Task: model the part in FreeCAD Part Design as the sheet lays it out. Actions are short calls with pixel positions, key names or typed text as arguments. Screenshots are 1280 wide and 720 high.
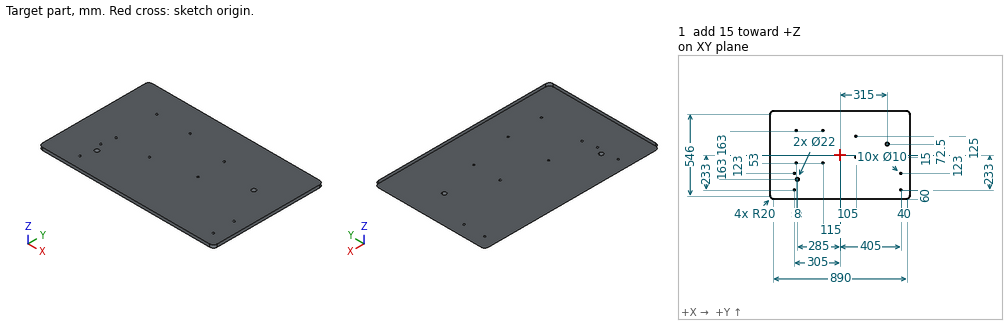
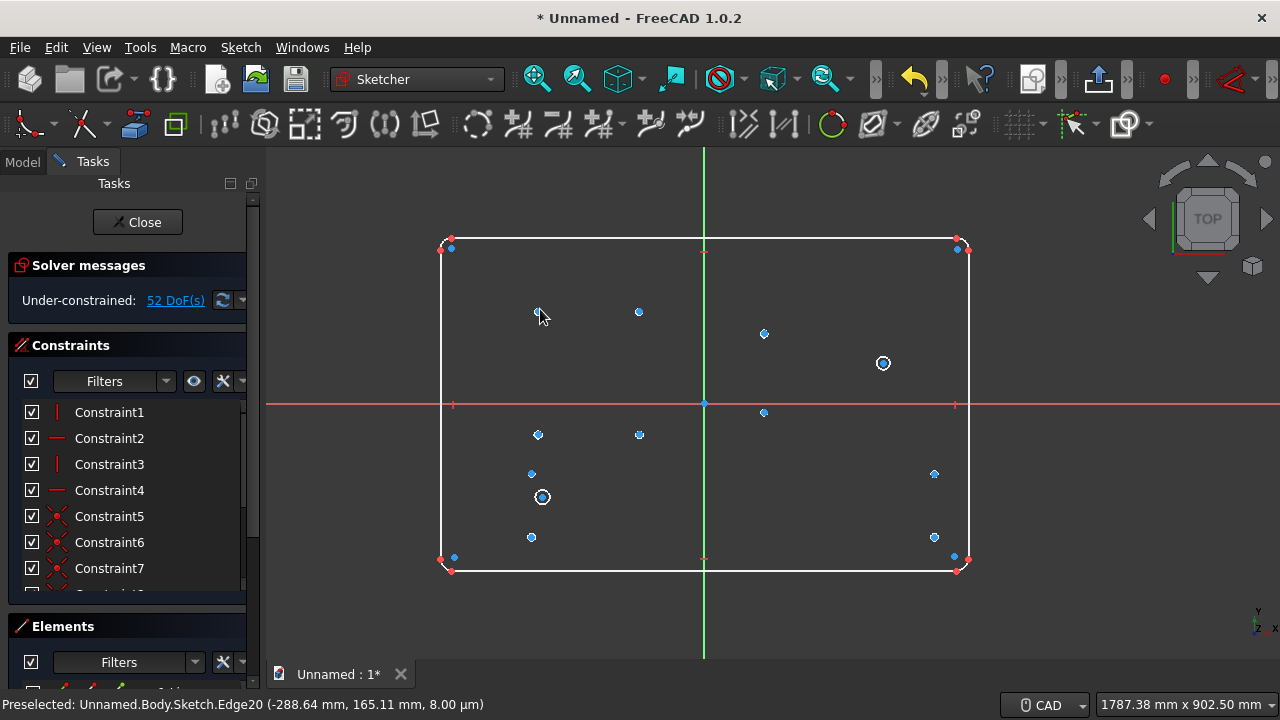
click(441, 343)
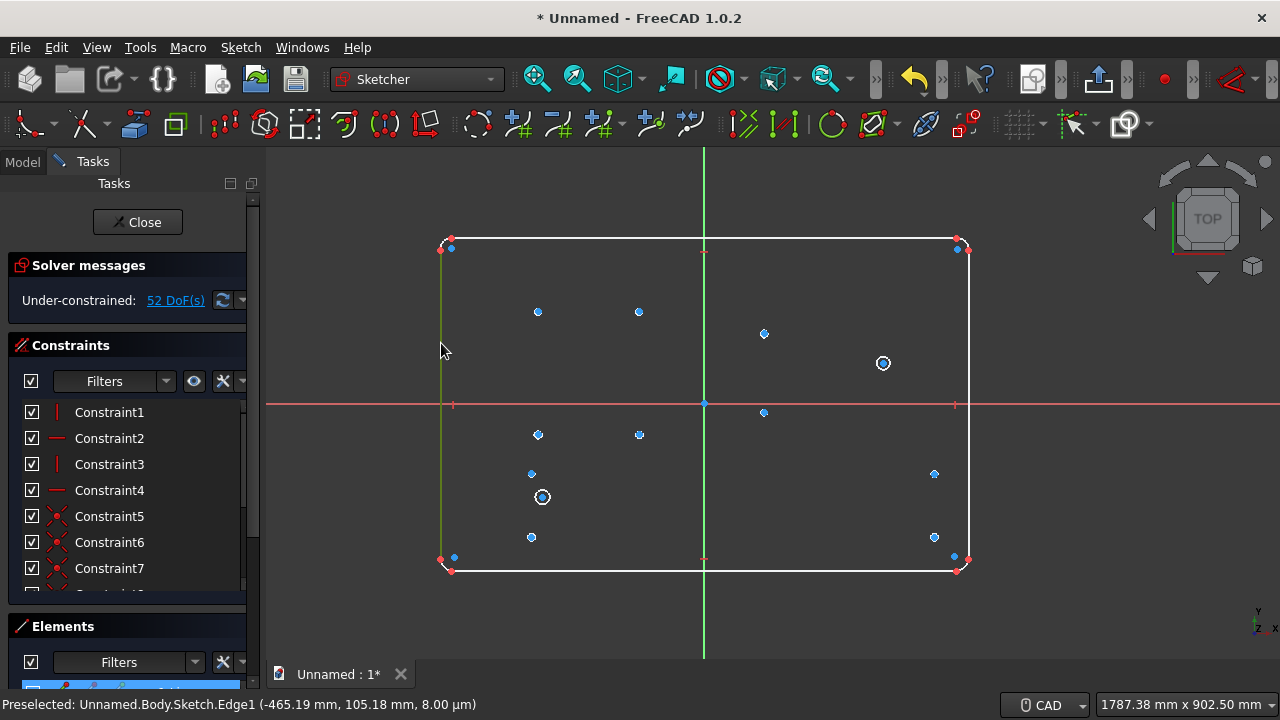
scroll(444, 567, up, 3)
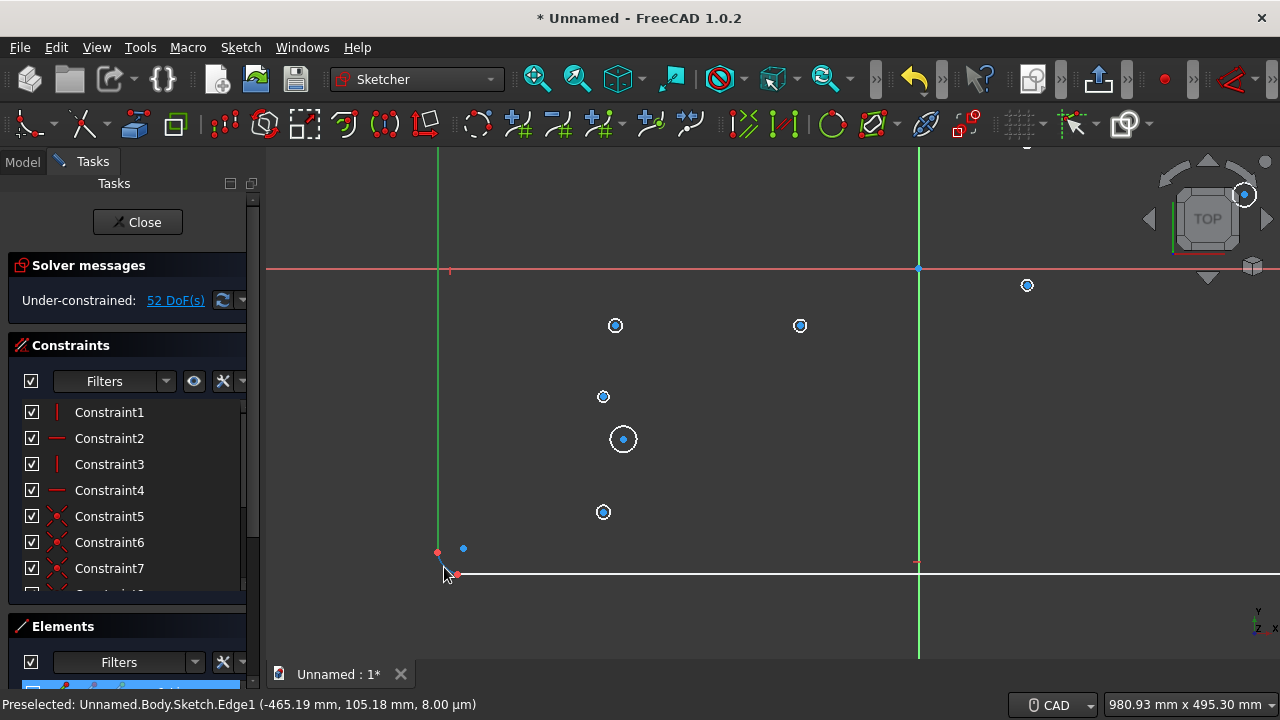
click(444, 566)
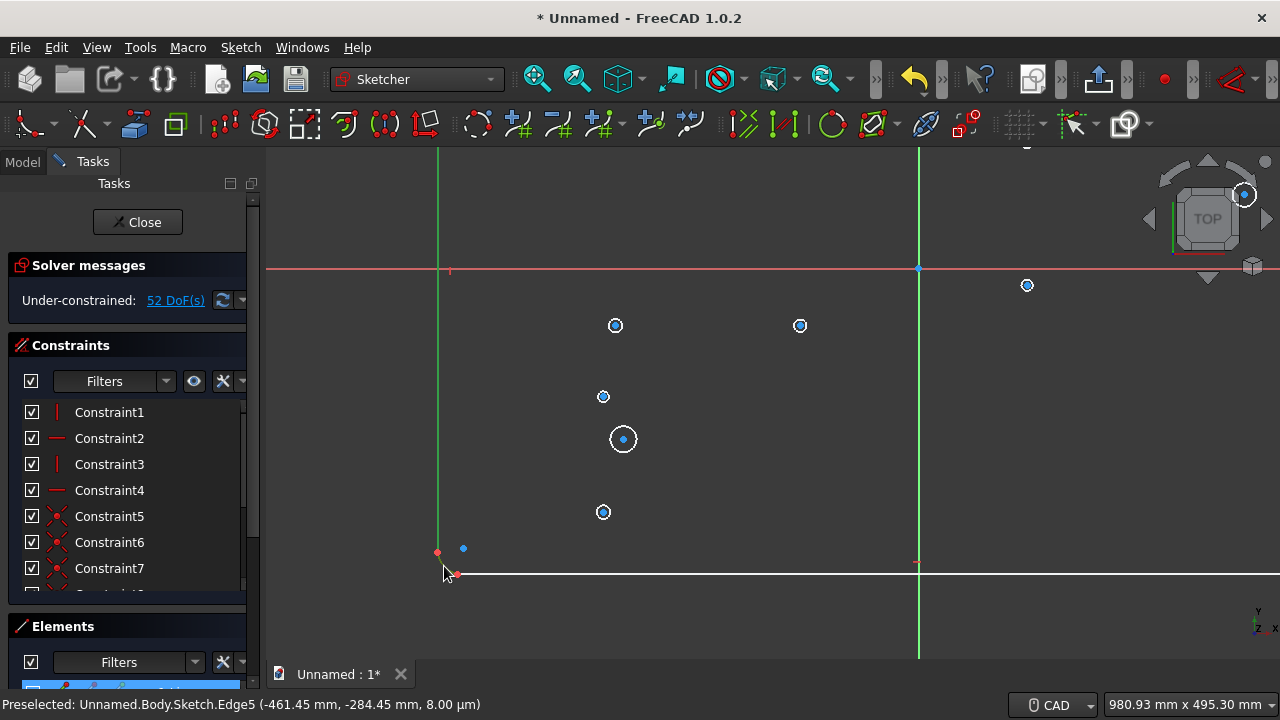
key(t)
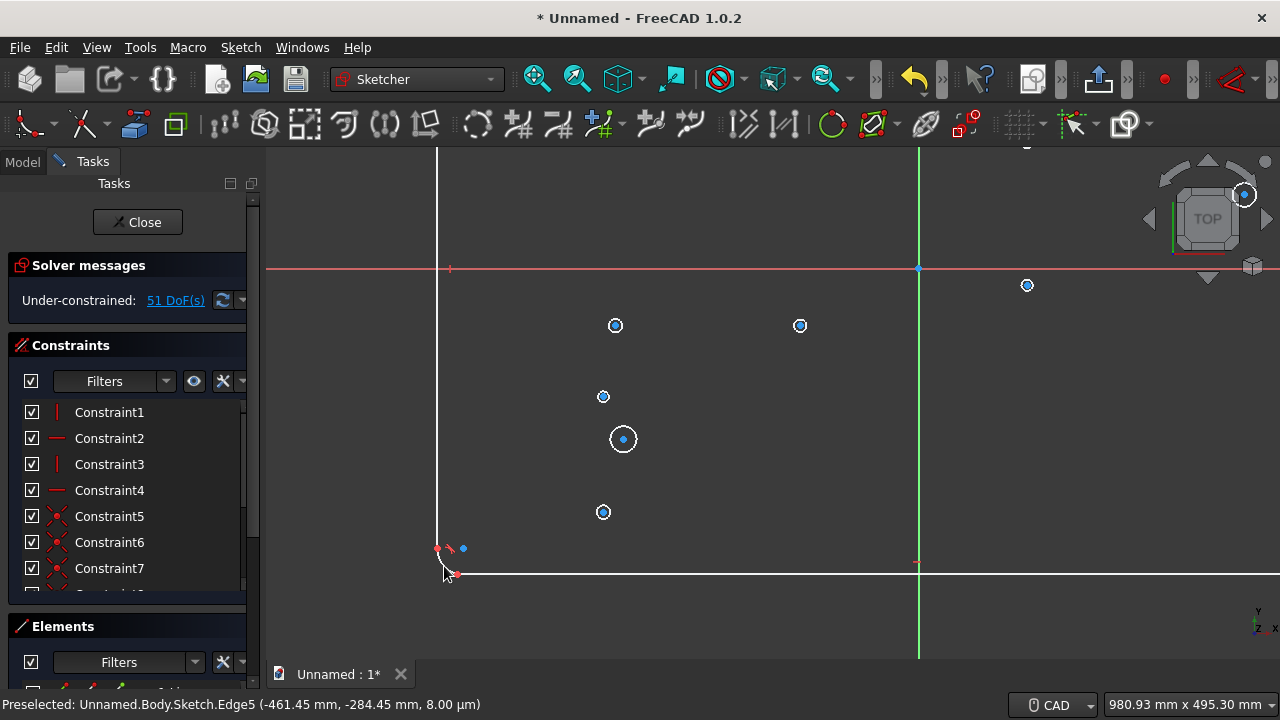
click(437, 381)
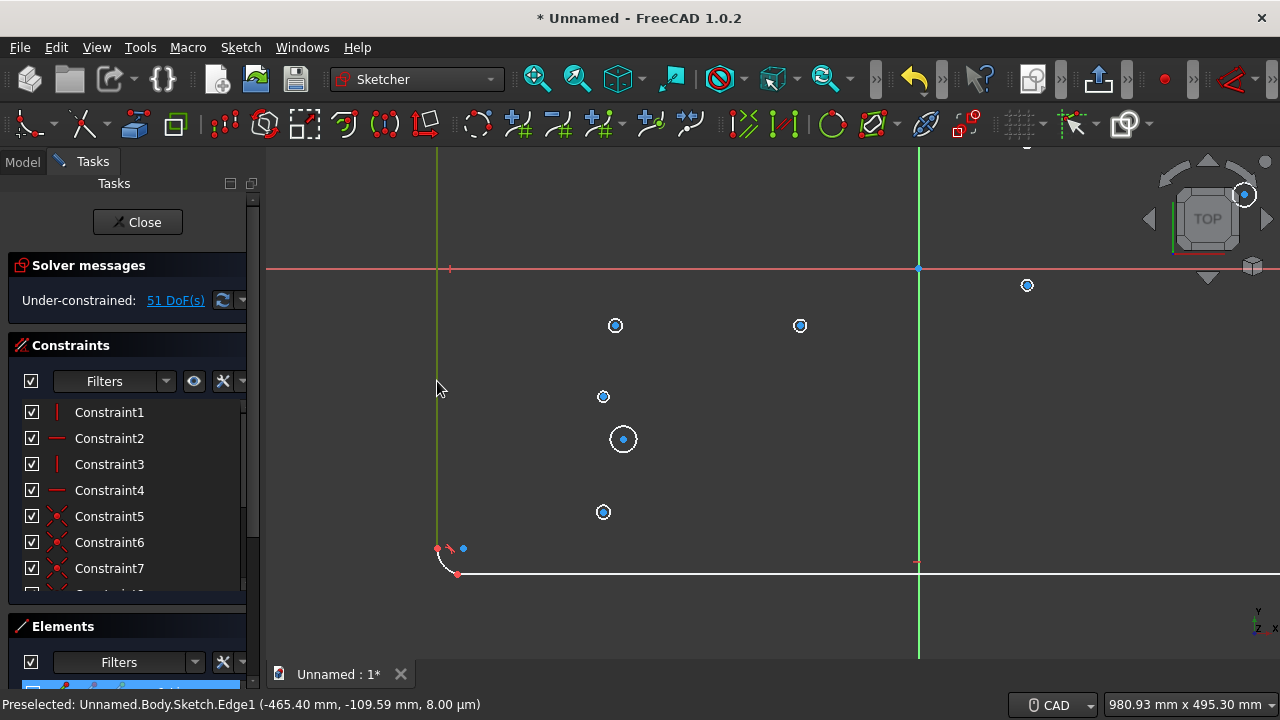
scroll(444, 566, down, 3)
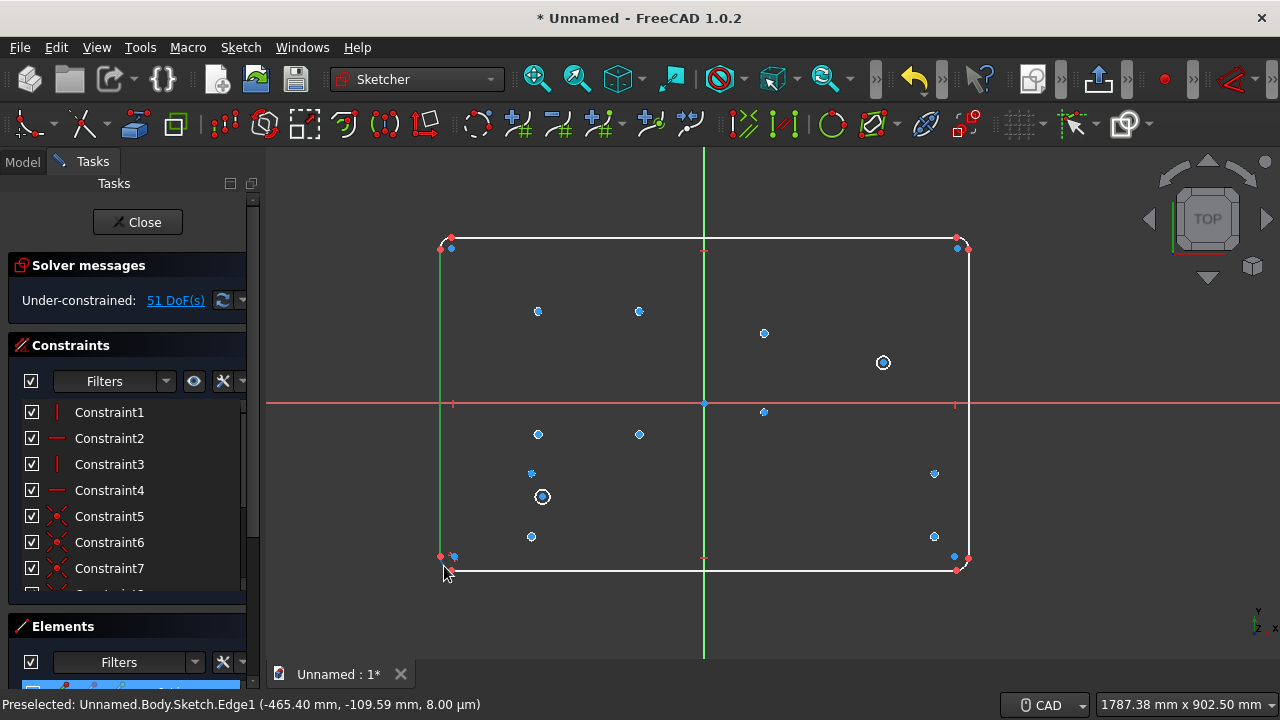
scroll(446, 239, up, 5)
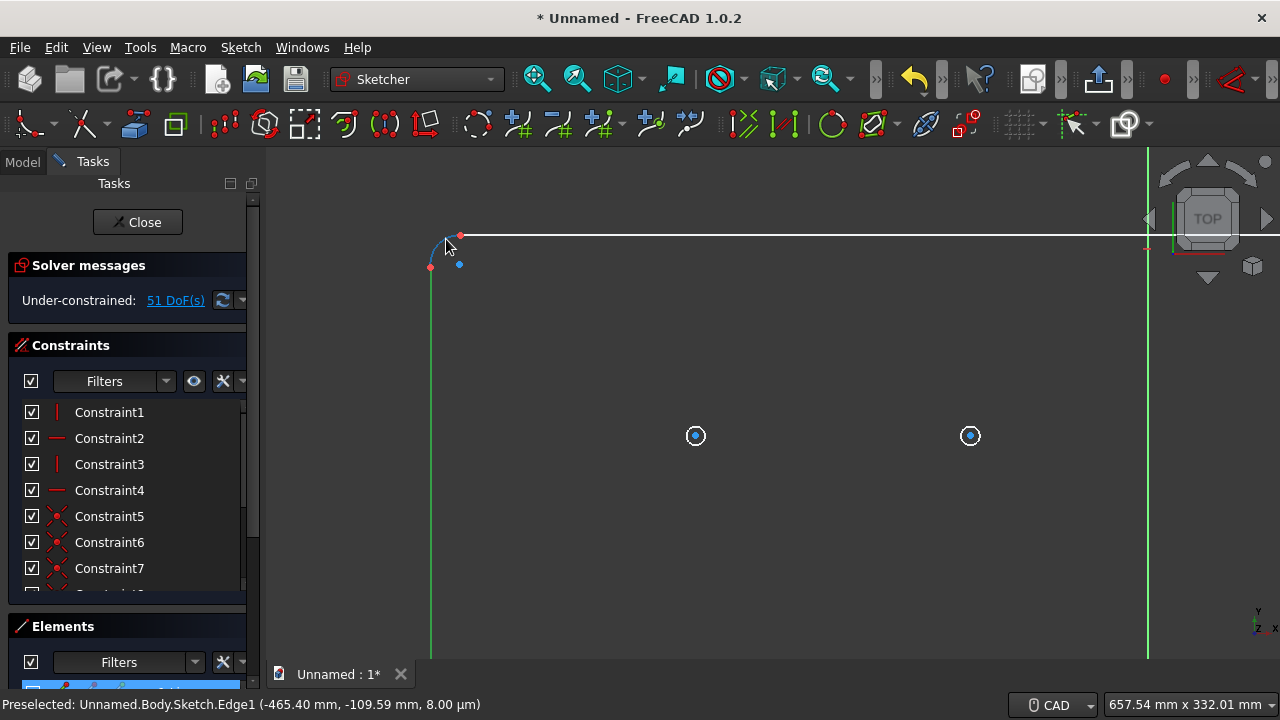
click(446, 239)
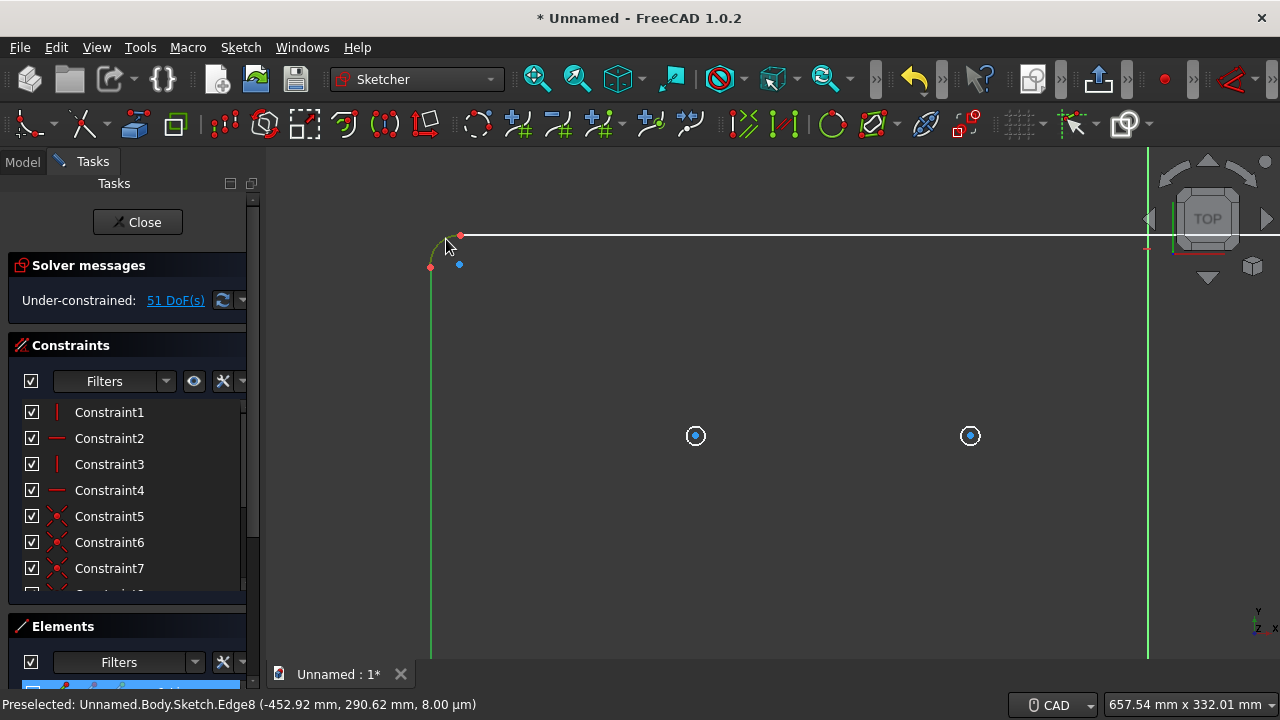
key(t)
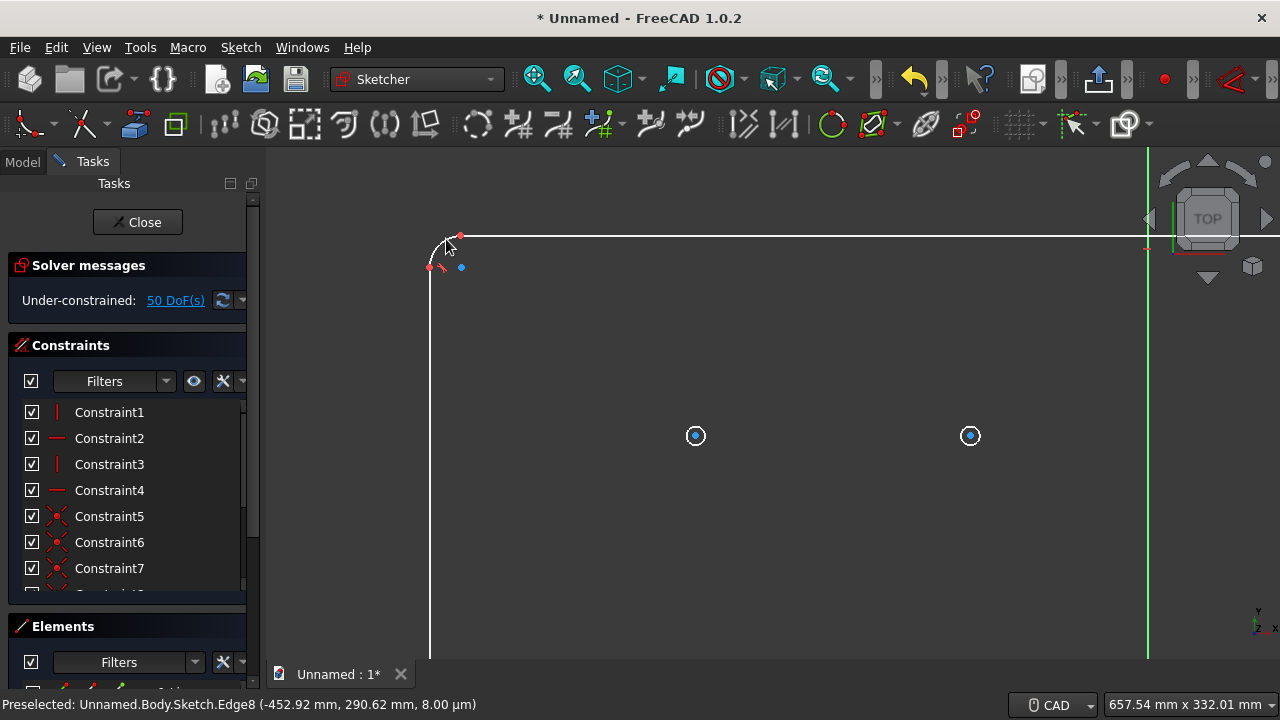
scroll(446, 239, down, 5)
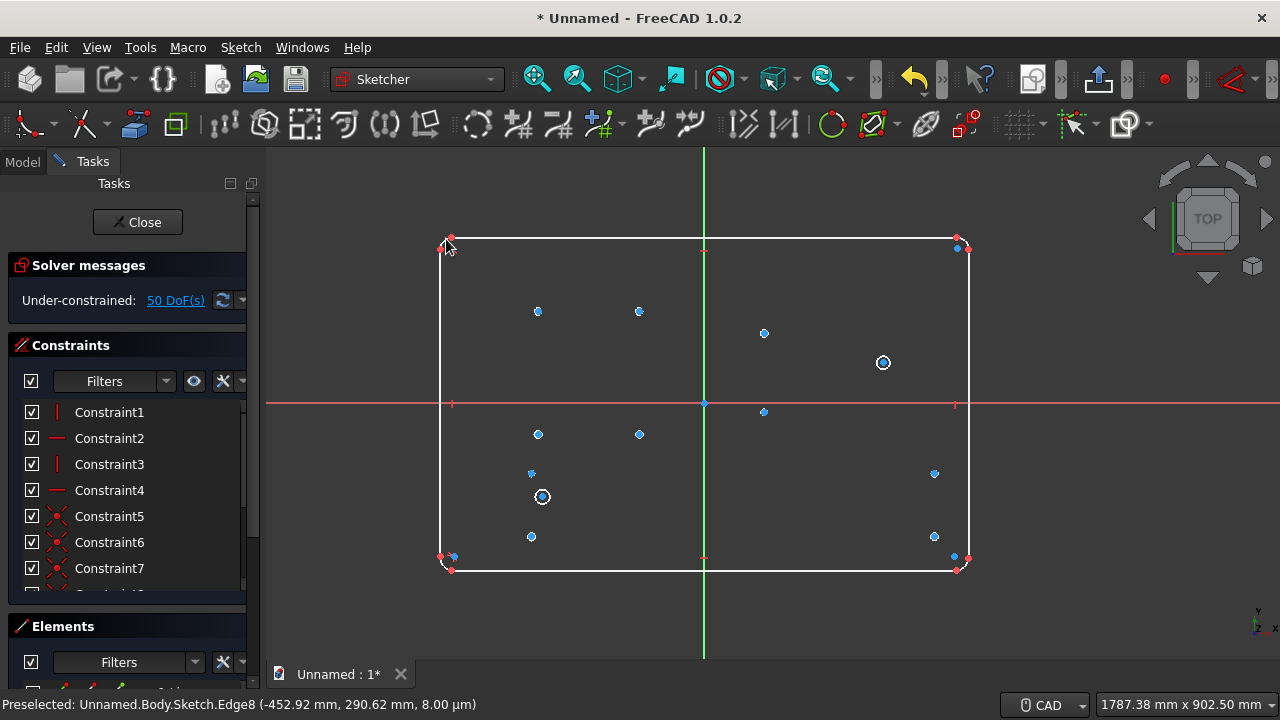
click(603, 571)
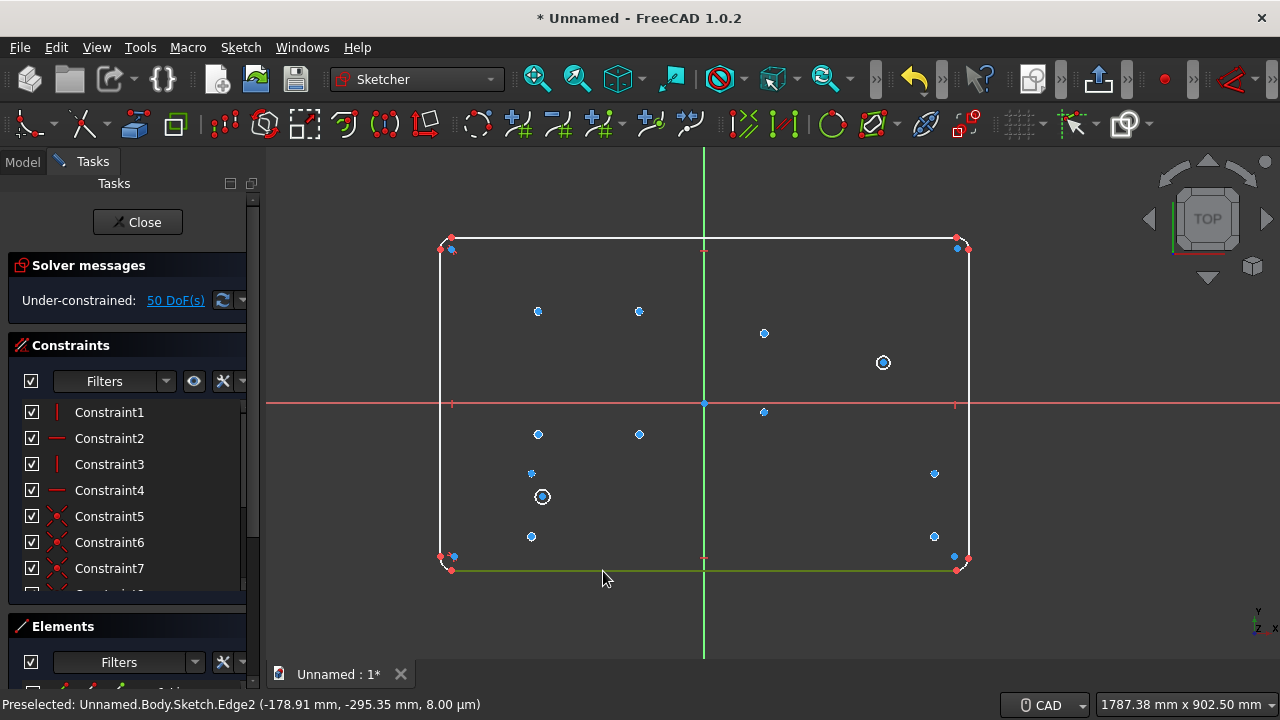
scroll(443, 566, up, 2)